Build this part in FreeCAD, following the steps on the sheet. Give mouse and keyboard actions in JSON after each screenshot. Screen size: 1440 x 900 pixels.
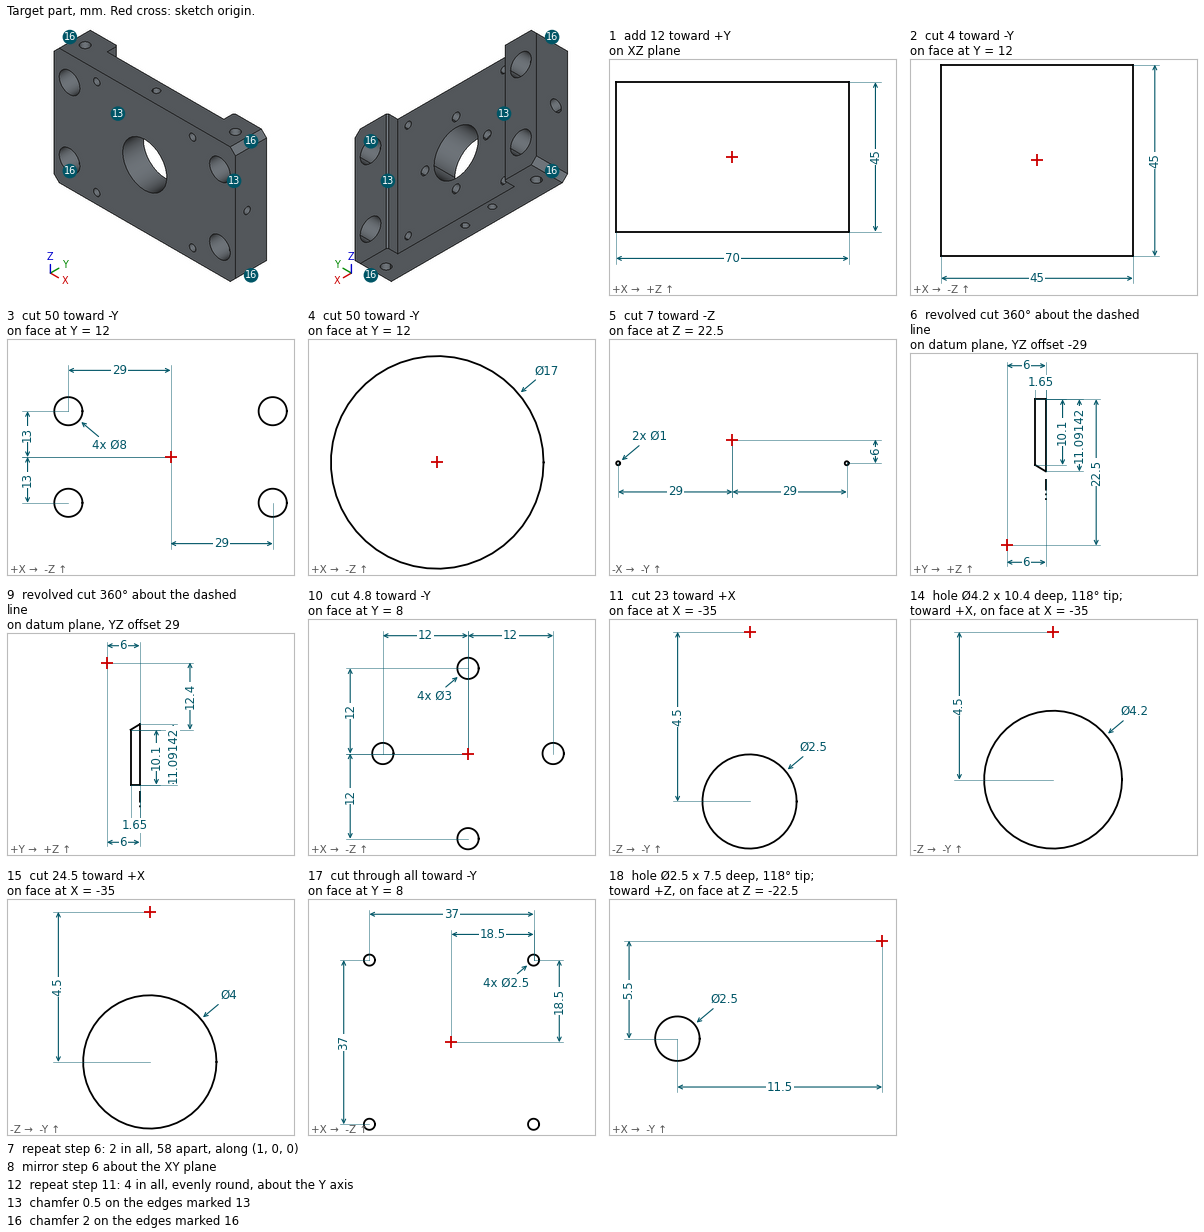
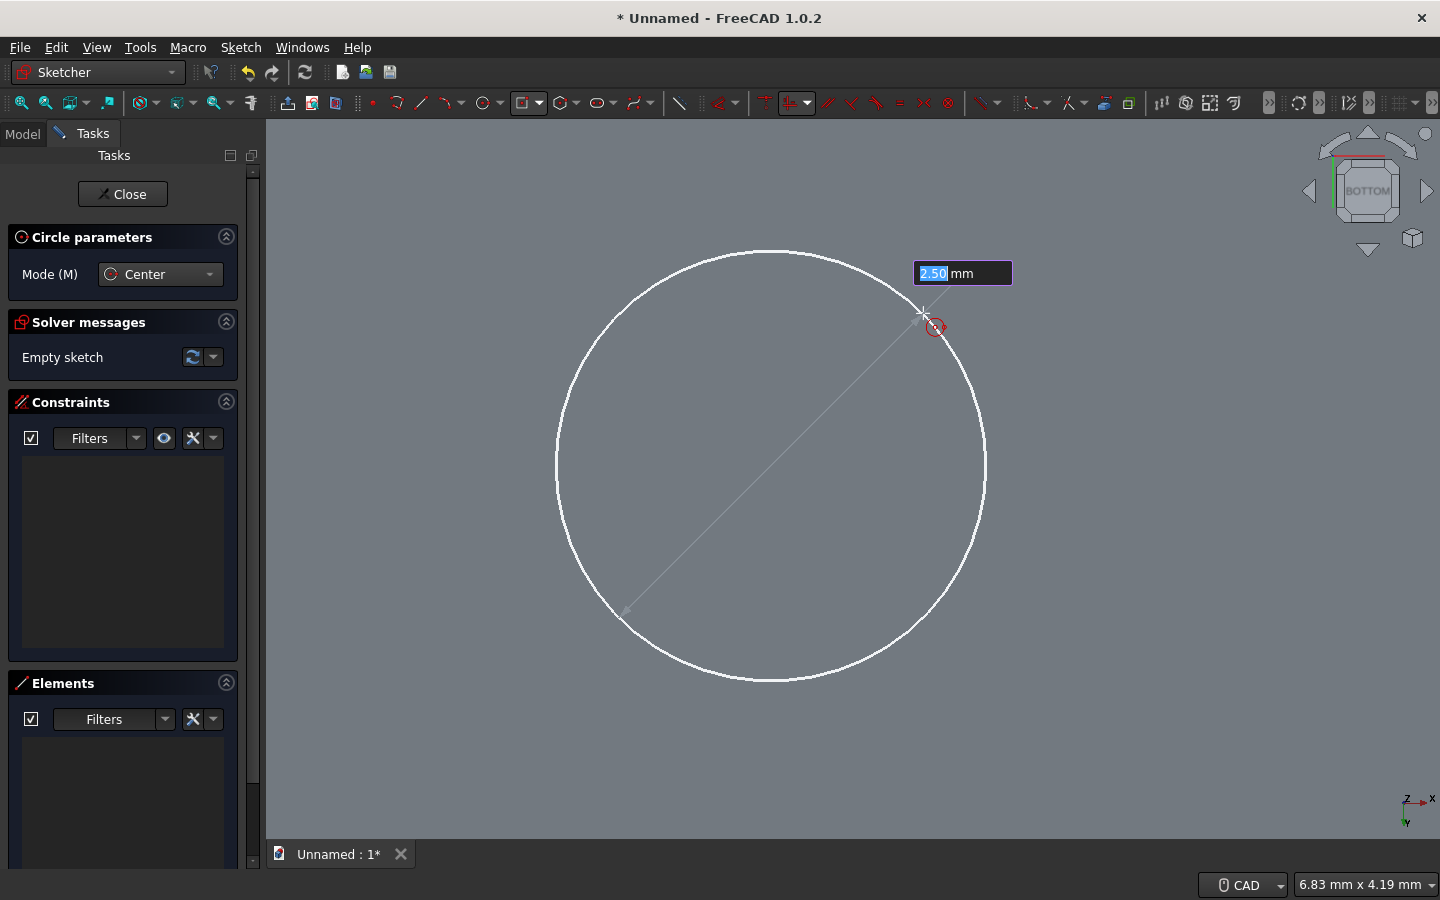
{"action": "type", "text": "2.5"}
{"action": "key", "text": "Return"}
{"action": "key", "text": "Escape"}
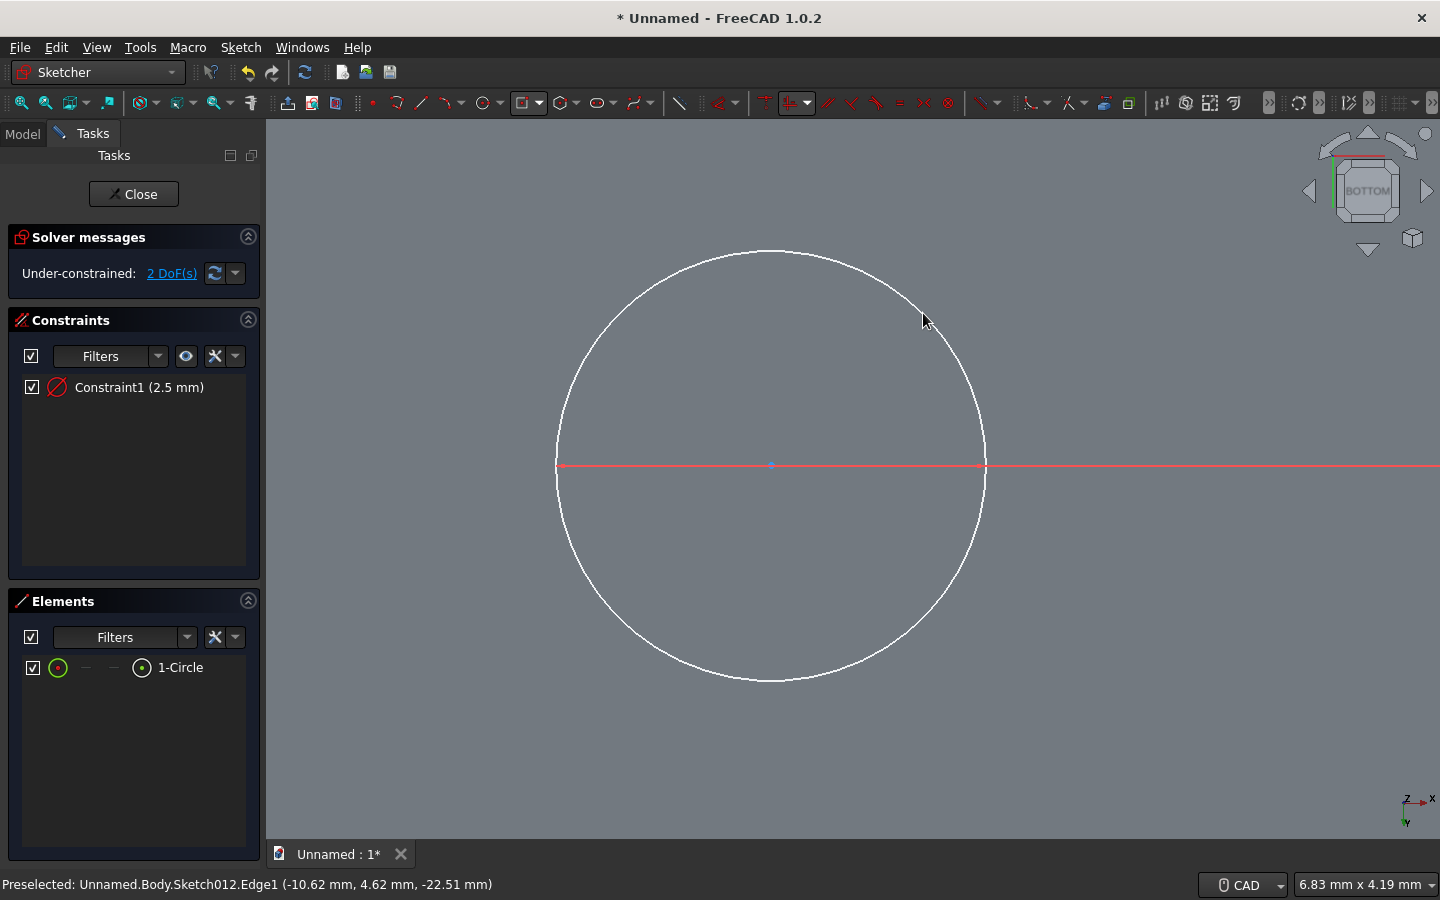
{"action": "left_click", "coordinate": [718, 104]}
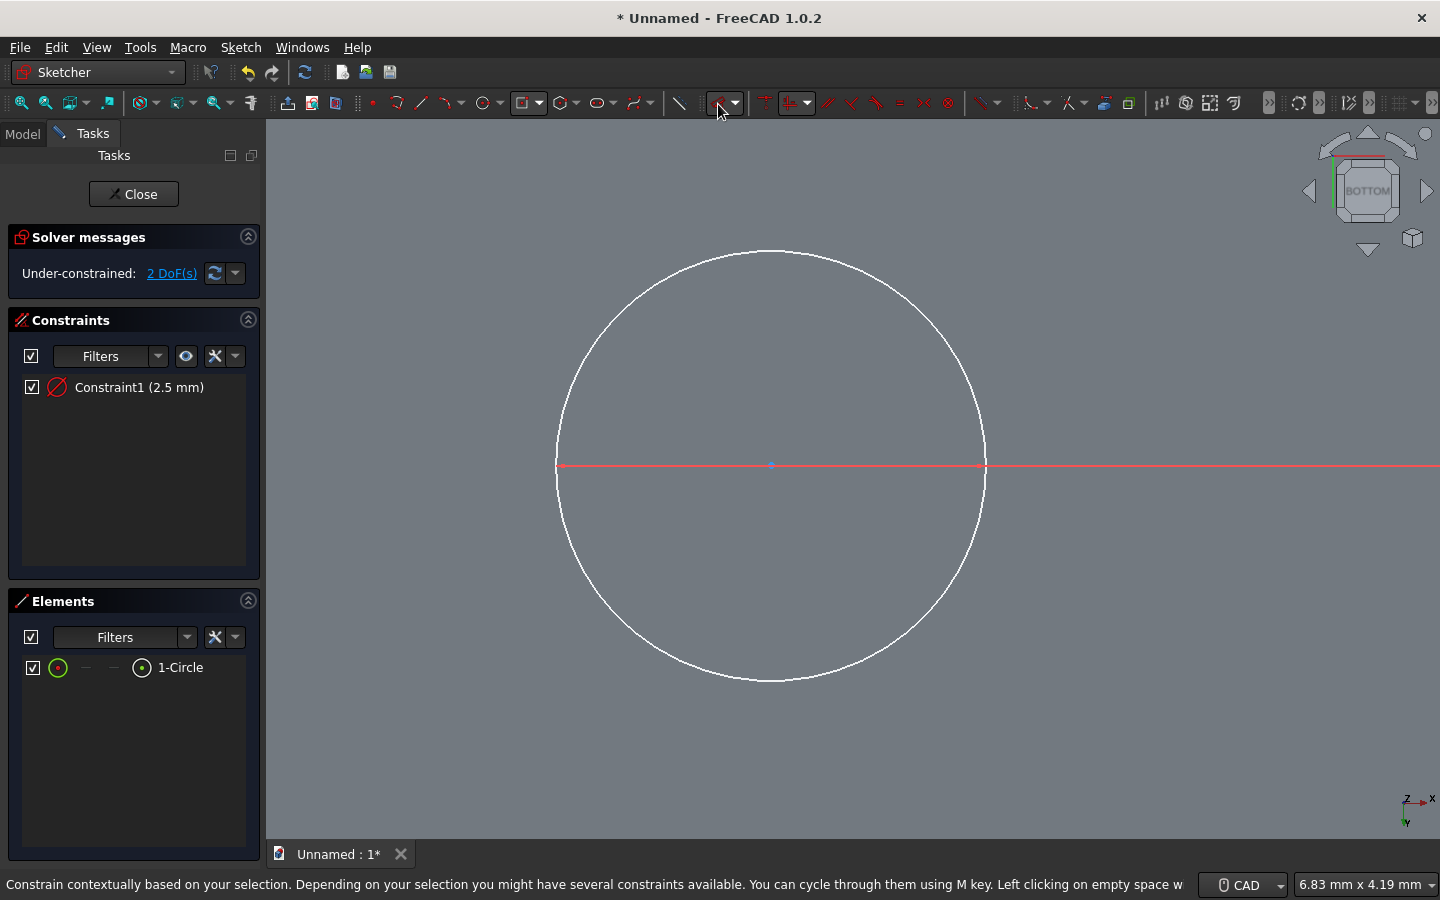
{"action": "left_click", "coordinate": [771, 466]}
{"action": "left_click", "coordinate": [737, 306]}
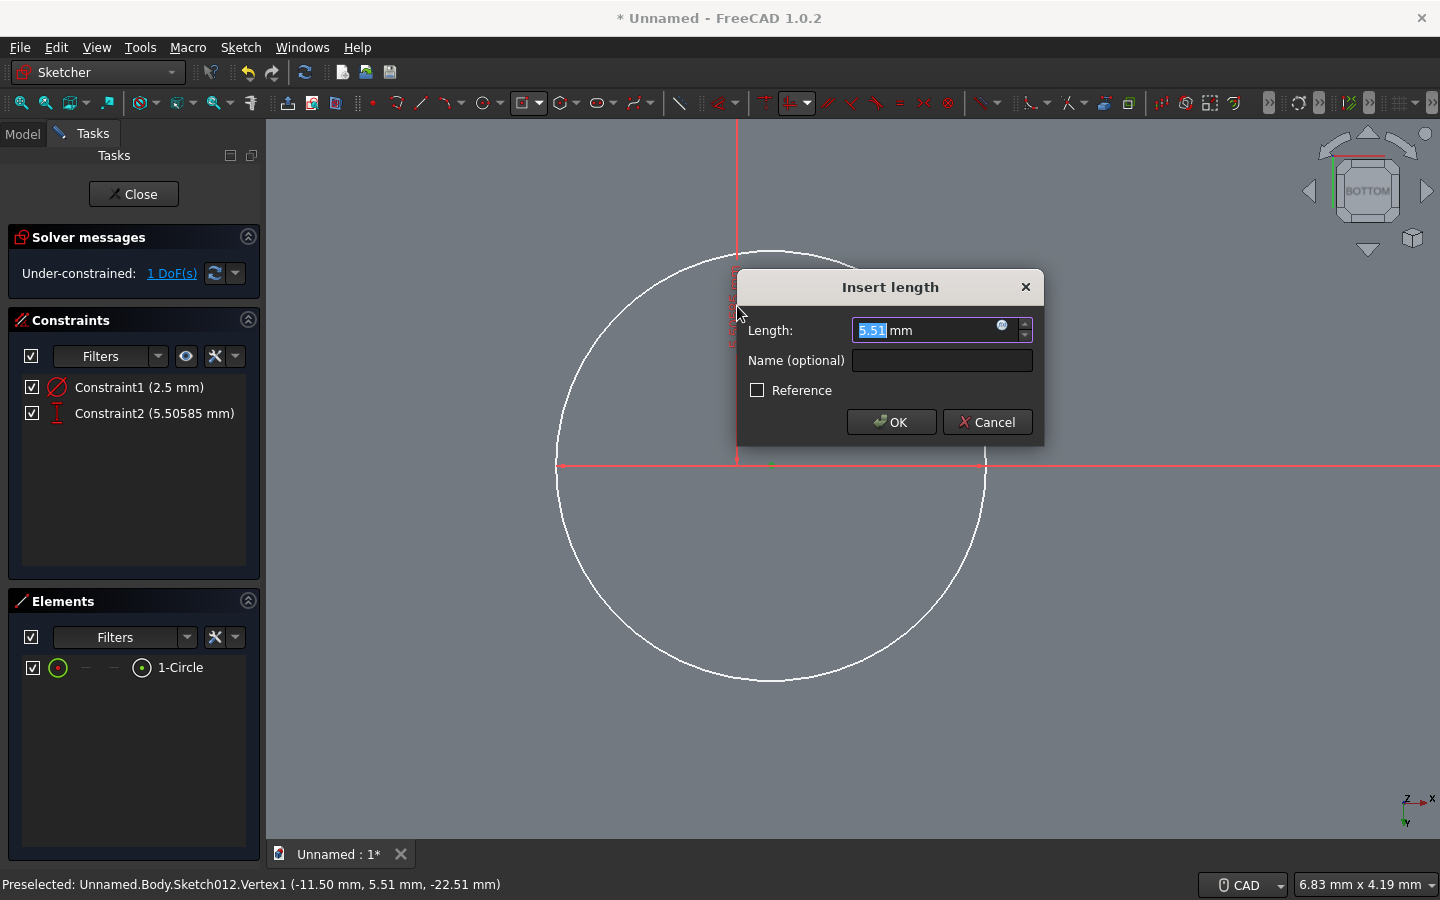
{"action": "type", "text": "5.5"}
{"action": "key", "text": "Return"}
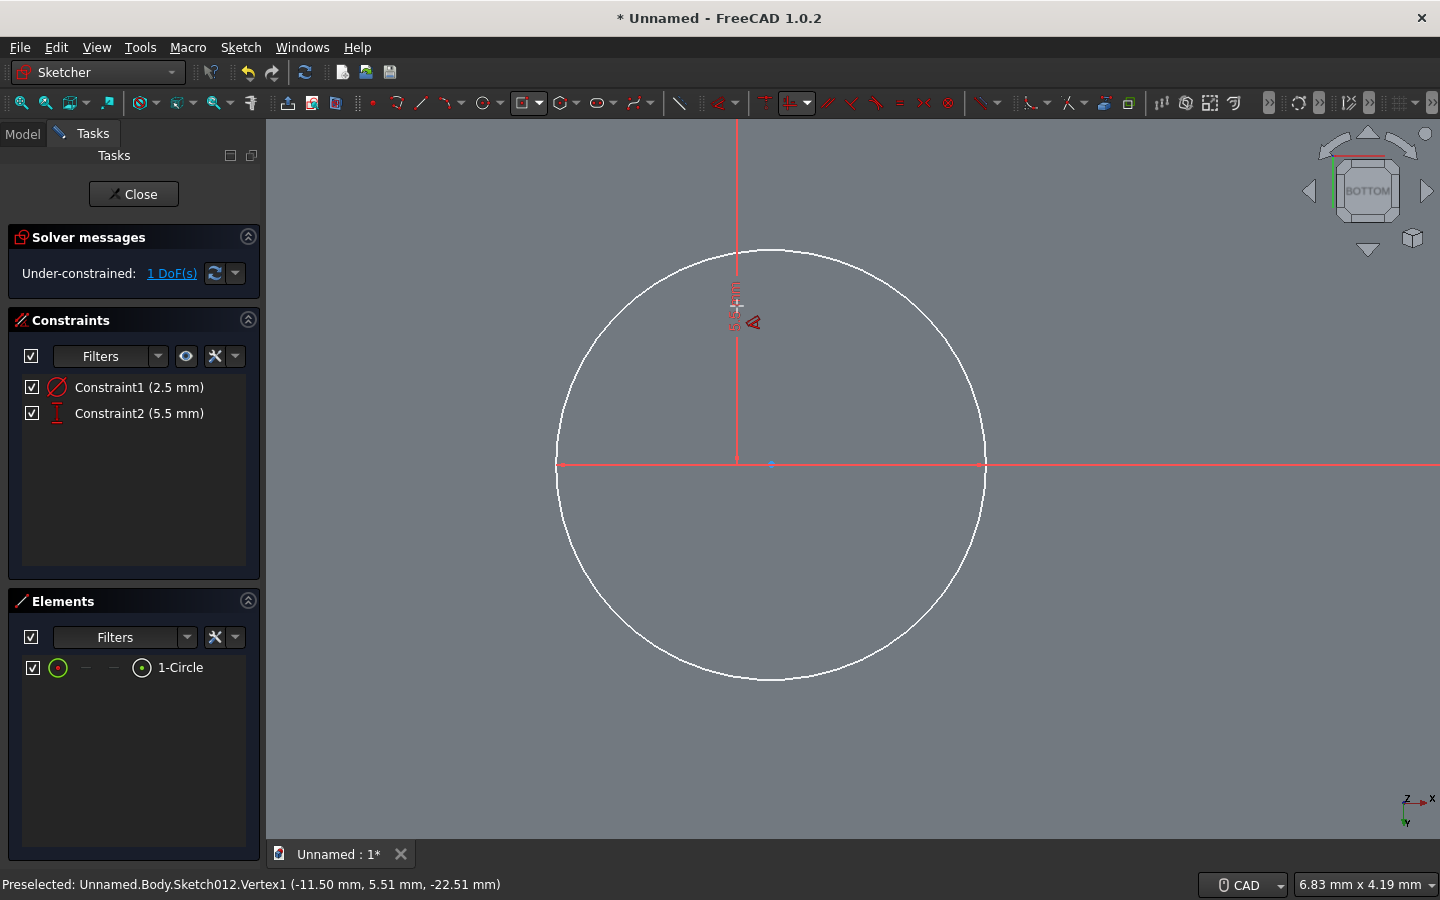
{"action": "left_click", "coordinate": [771, 465]}
{"action": "left_click", "coordinate": [1023, 499]}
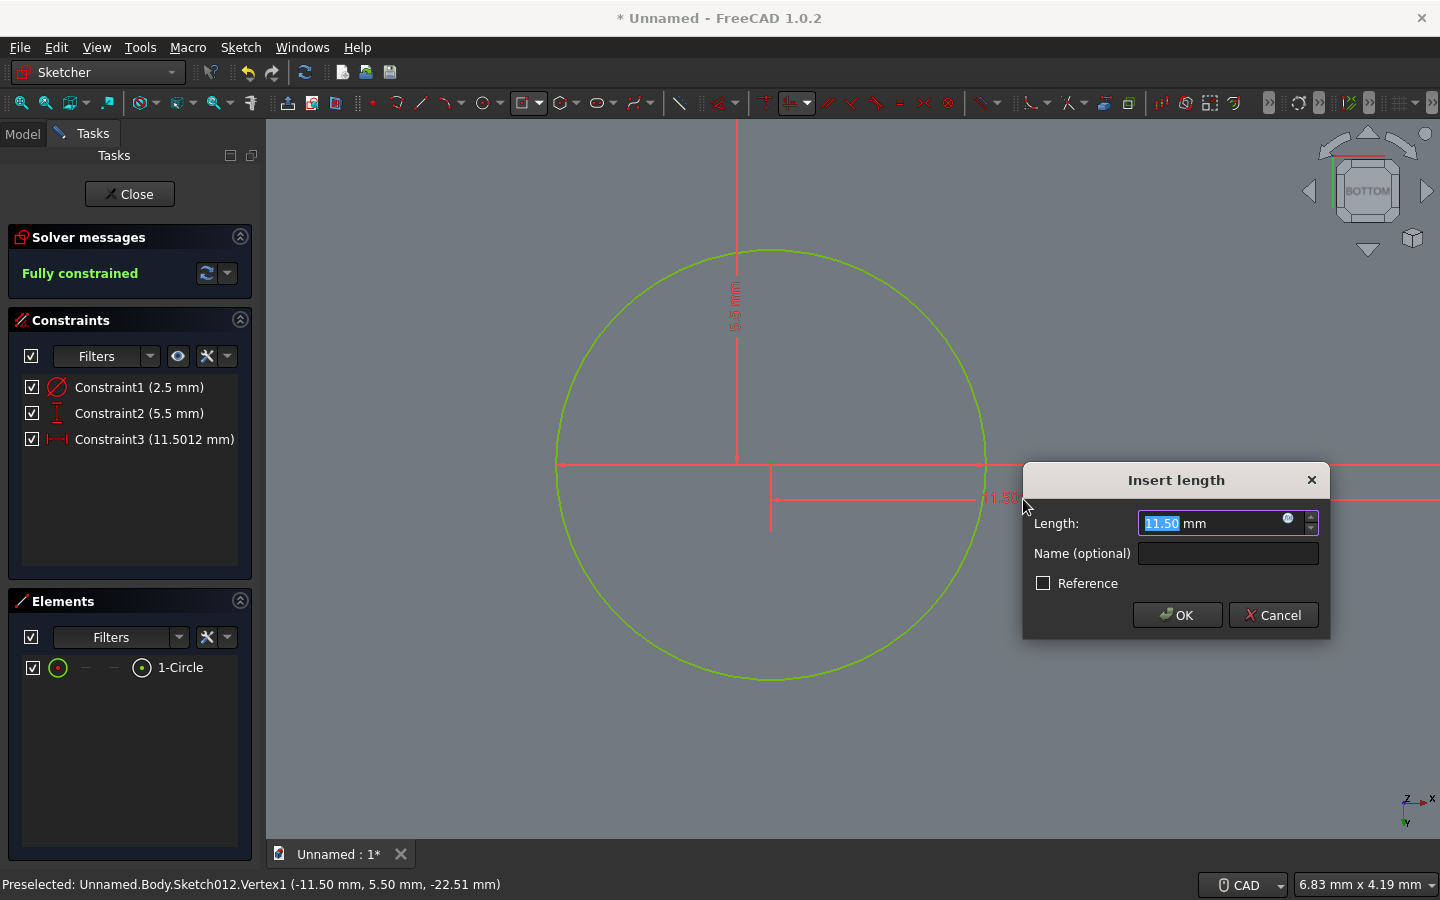
{"action": "type", "text": "11.5"}
{"action": "key", "text": "Return"}
{"action": "key", "text": "Escape"}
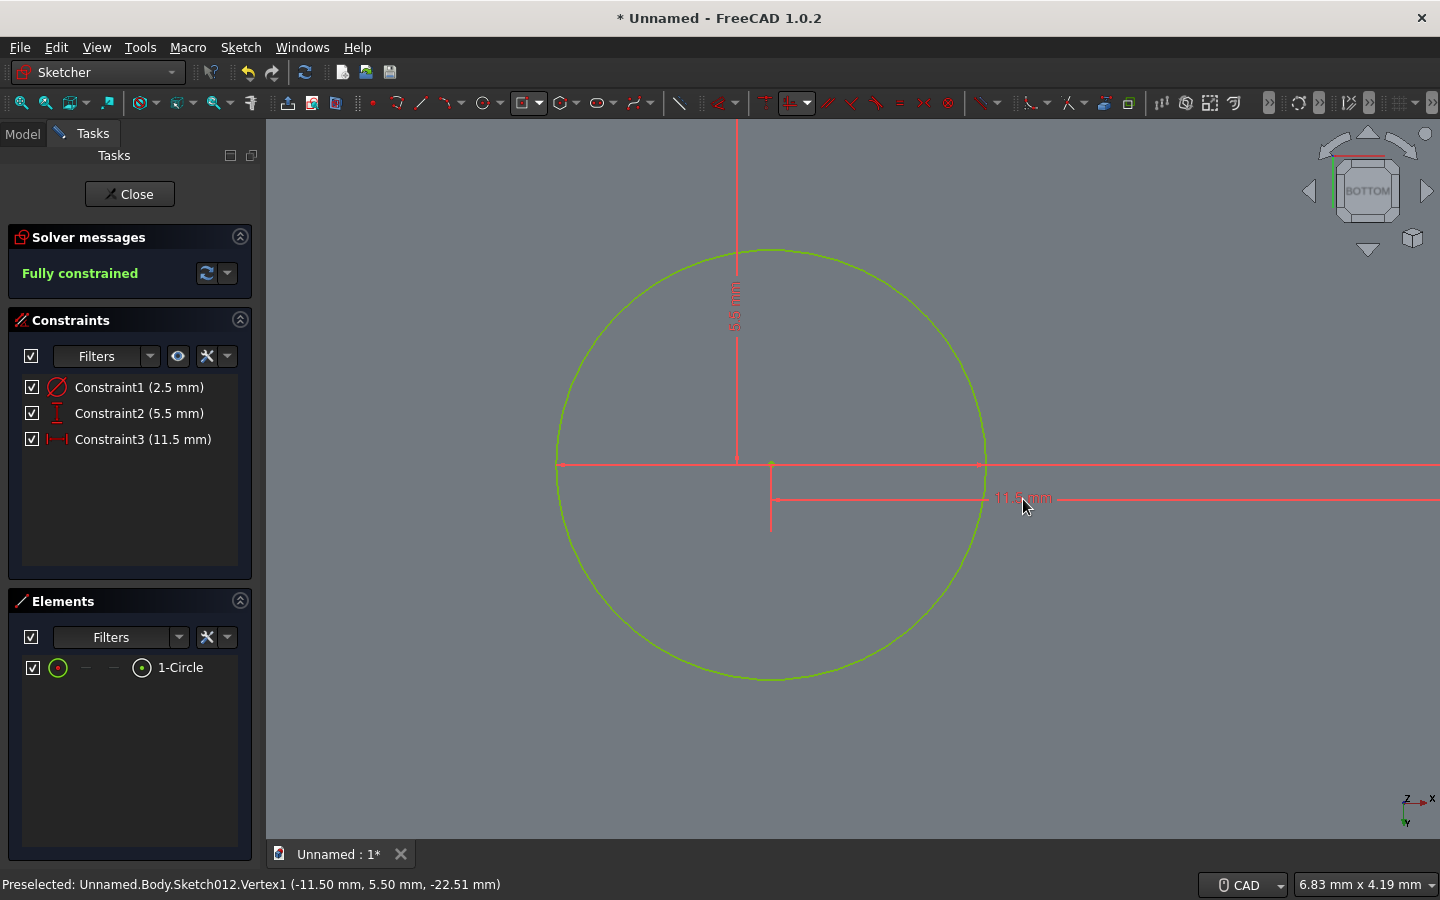
{"action": "left_click", "coordinate": [130, 194]}